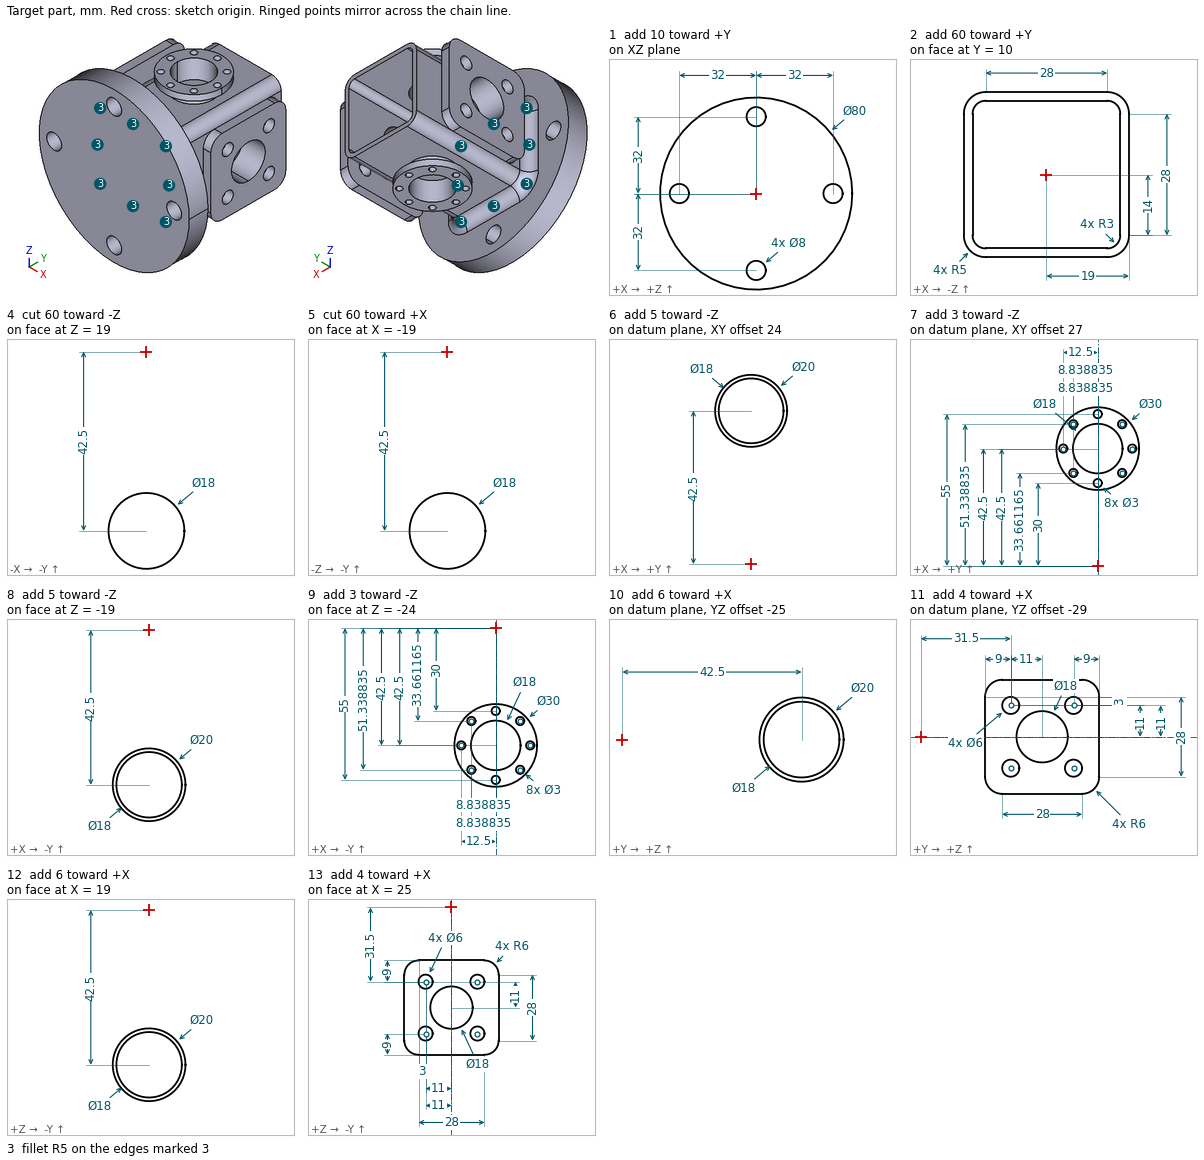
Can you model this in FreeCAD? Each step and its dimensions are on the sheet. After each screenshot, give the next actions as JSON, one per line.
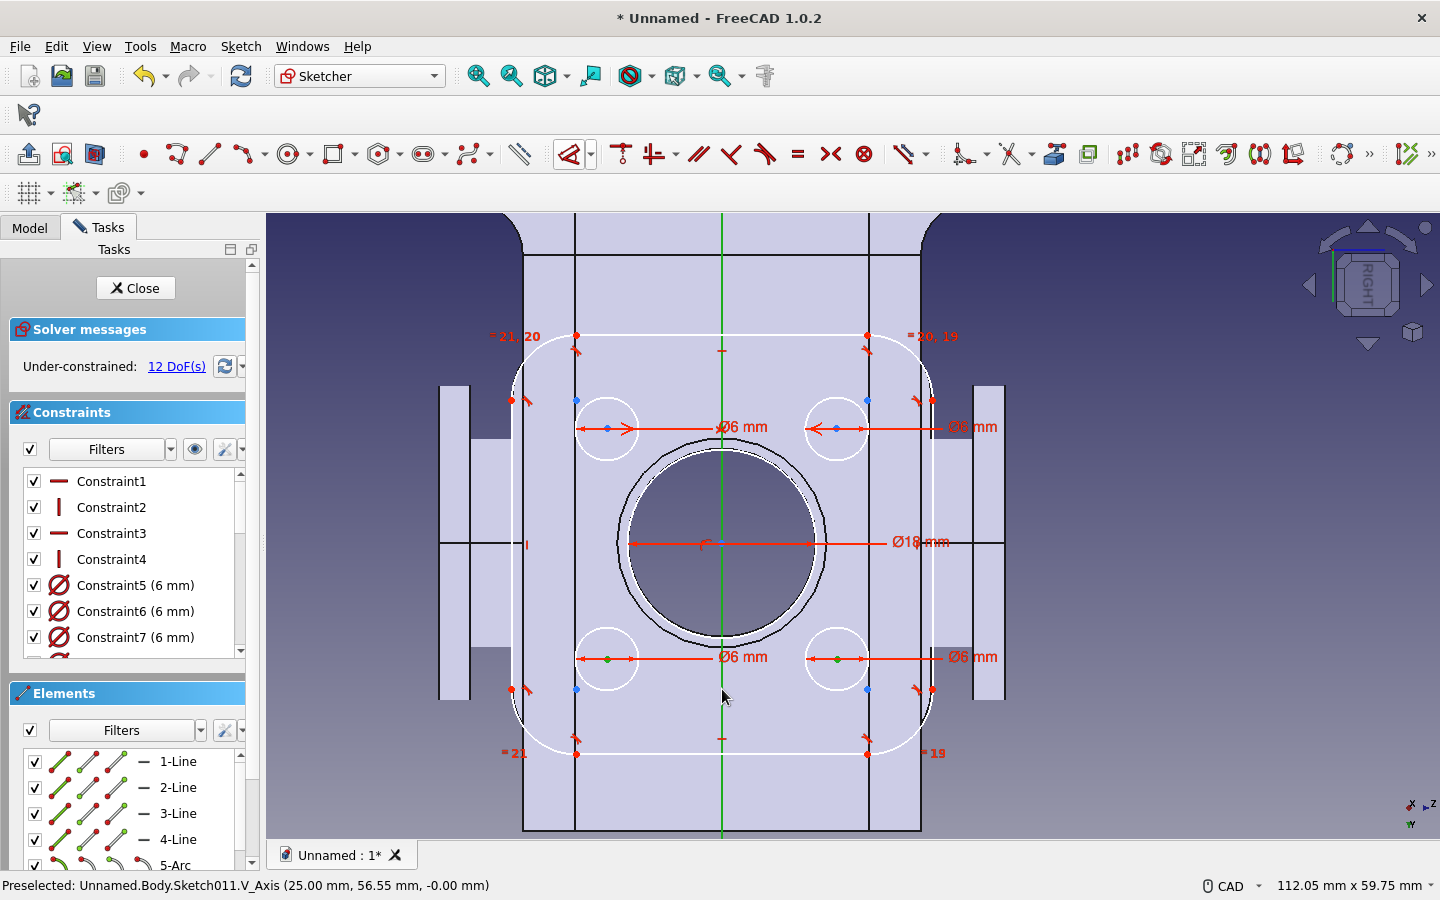
{"action": "left_click", "coordinate": [831, 154]}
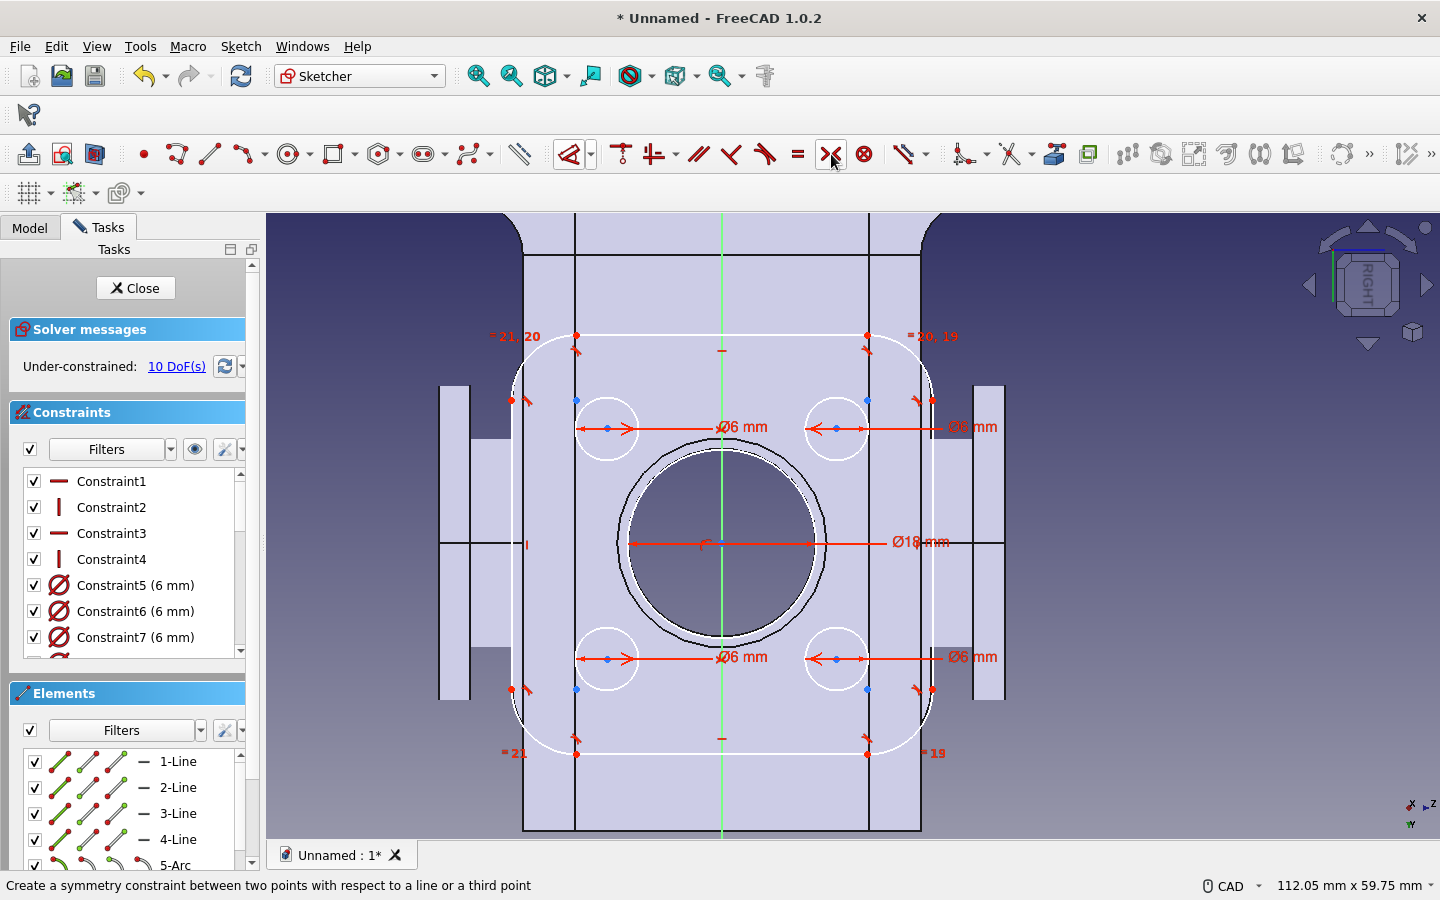
{"action": "left_click", "coordinate": [897, 747]}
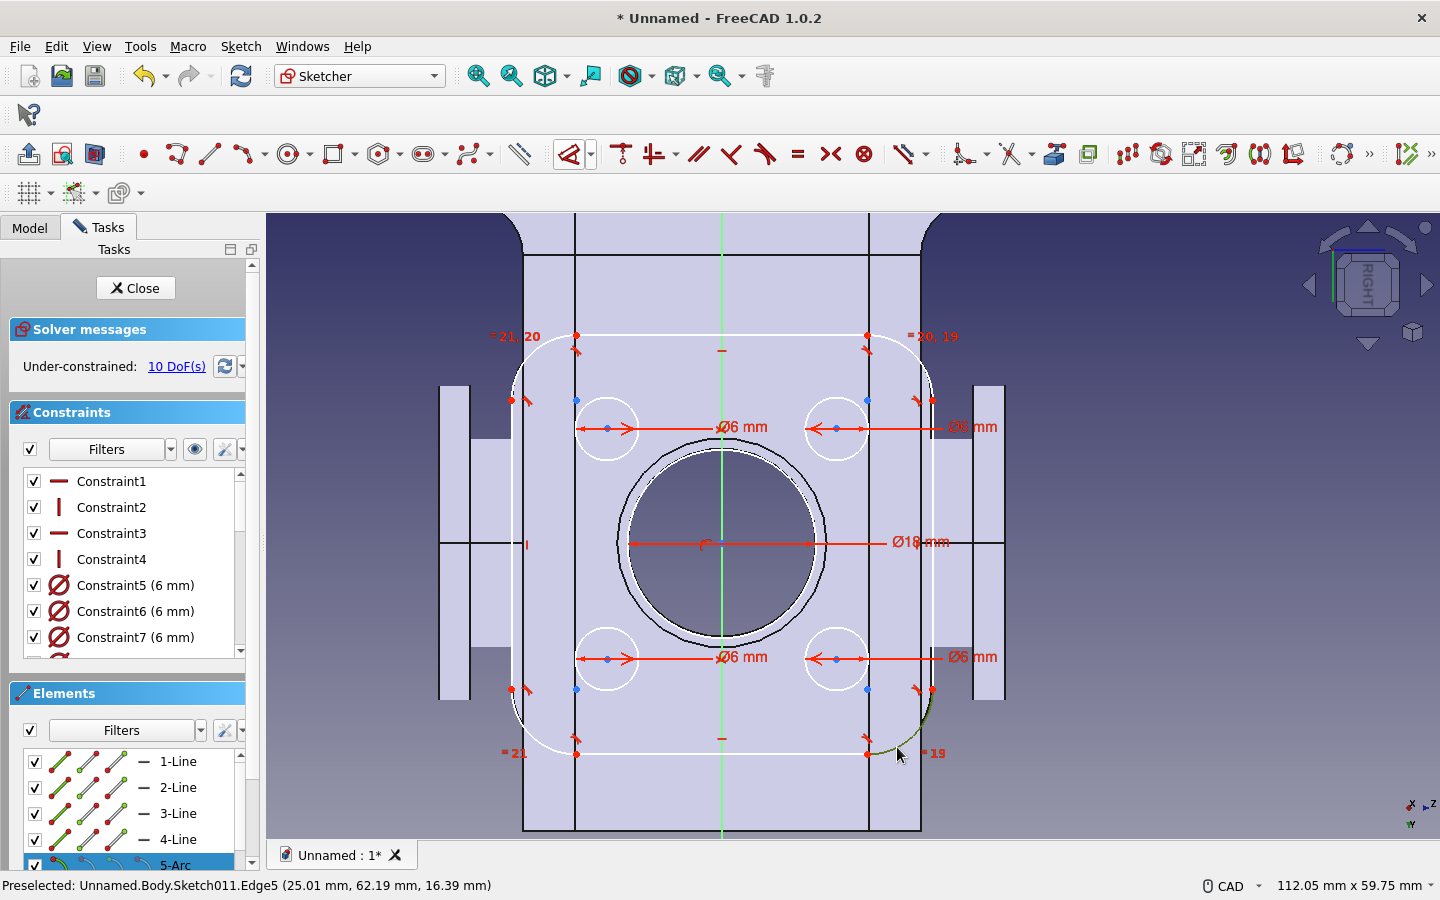
{"action": "key", "text": "k r"}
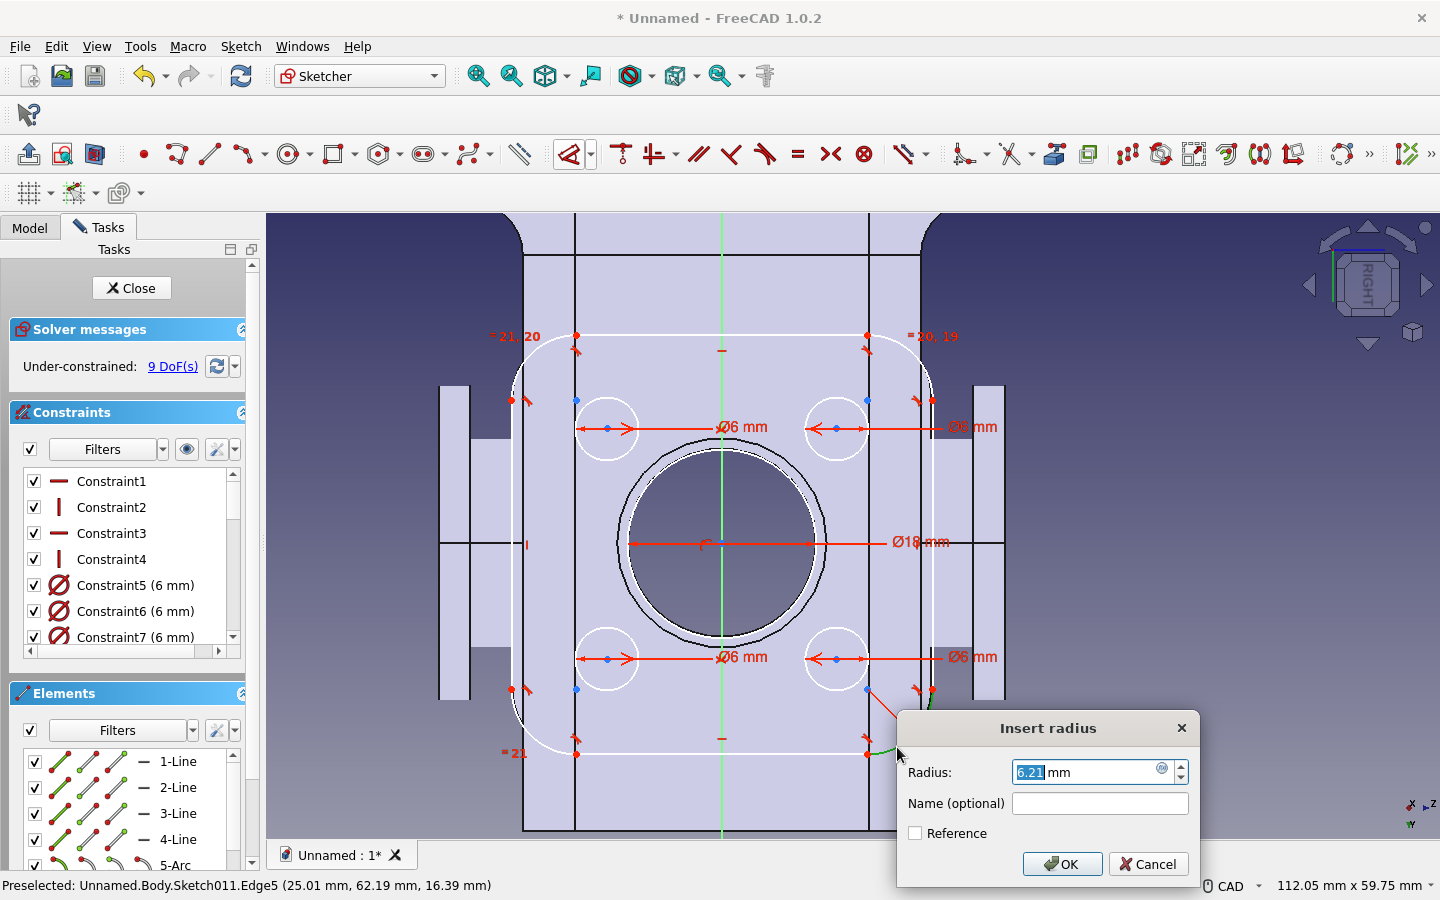
{"action": "type", "text": "6"}
{"action": "key", "text": "Return"}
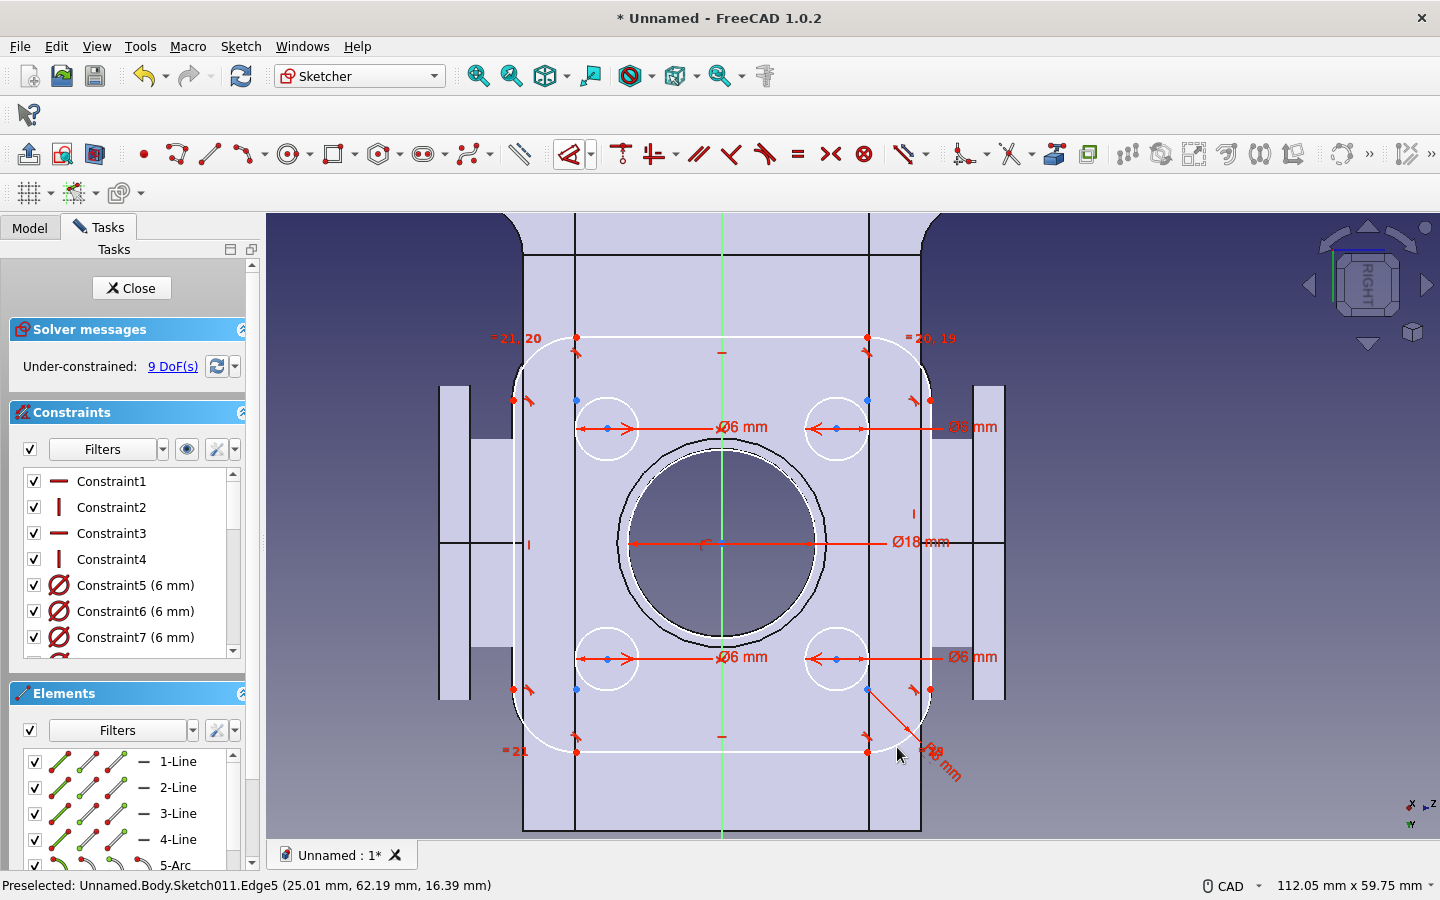
{"action": "left_click", "coordinate": [664, 752]}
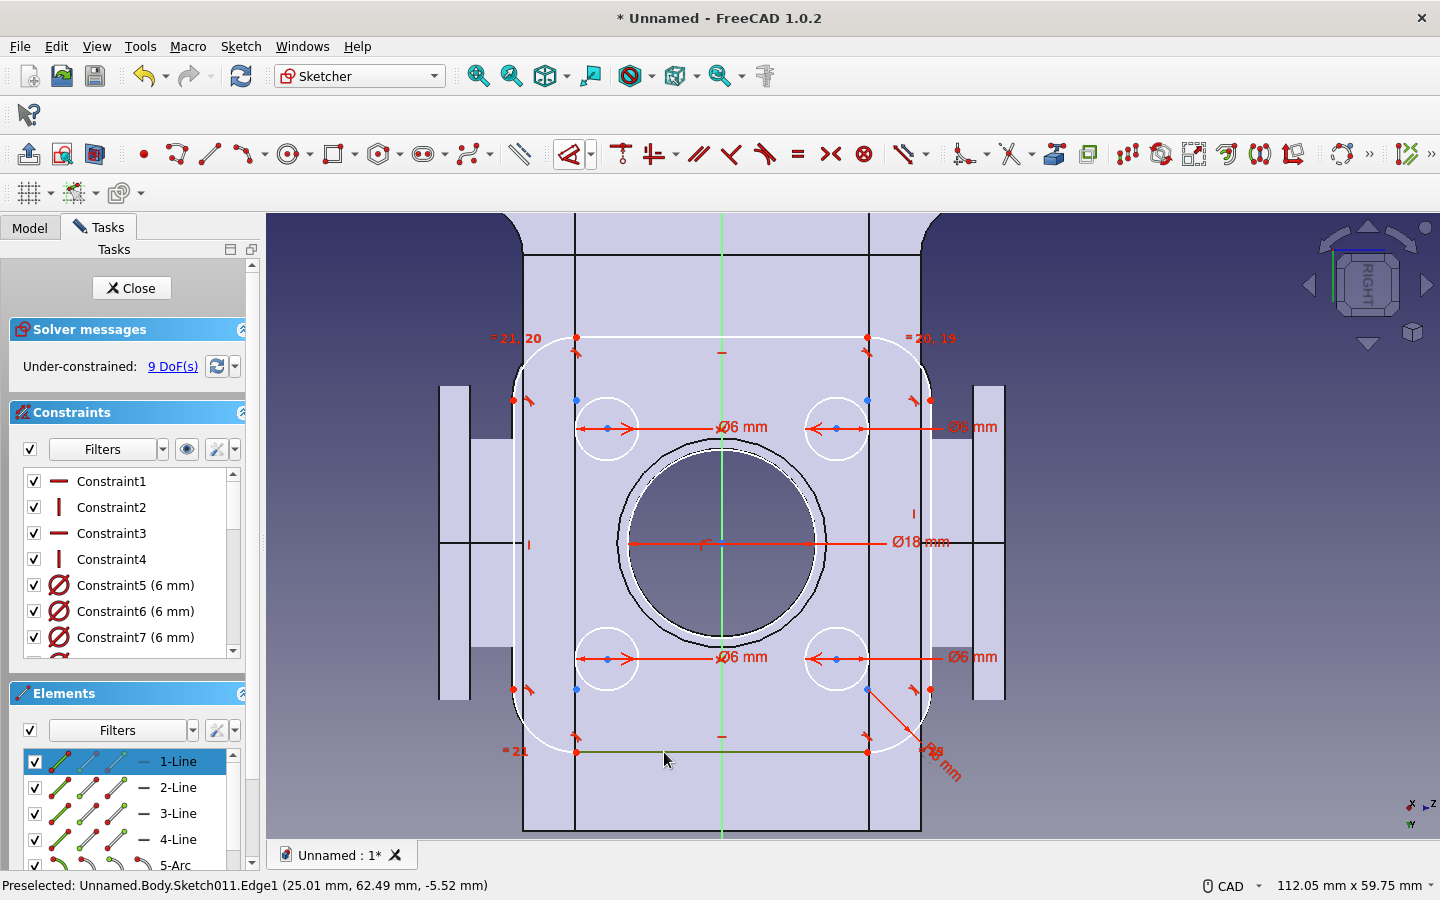
{"action": "left_click", "coordinate": [590, 154]}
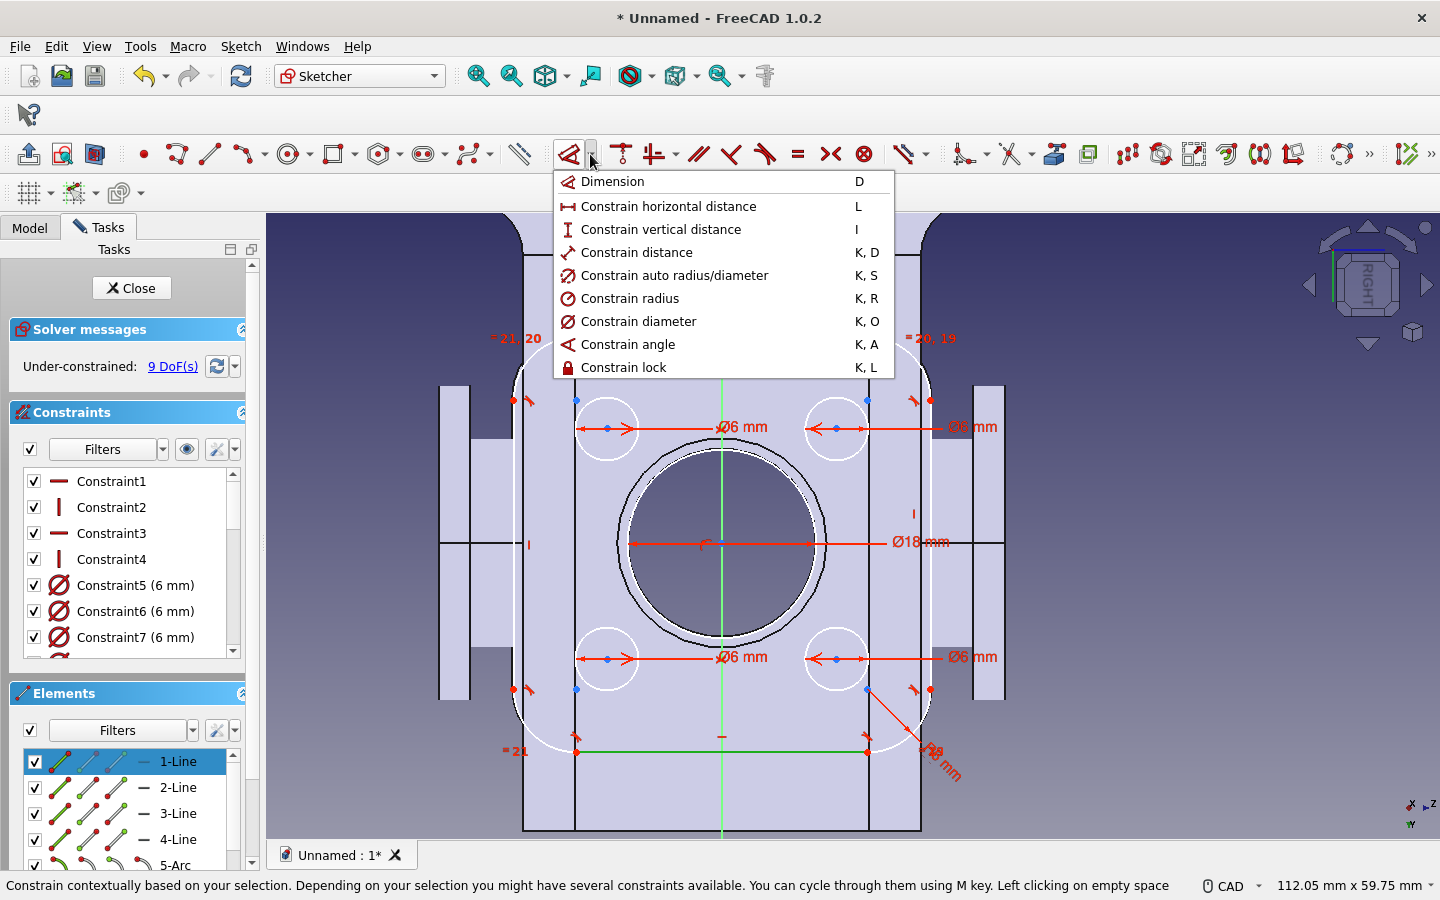
{"action": "left_click", "coordinate": [724, 206]}